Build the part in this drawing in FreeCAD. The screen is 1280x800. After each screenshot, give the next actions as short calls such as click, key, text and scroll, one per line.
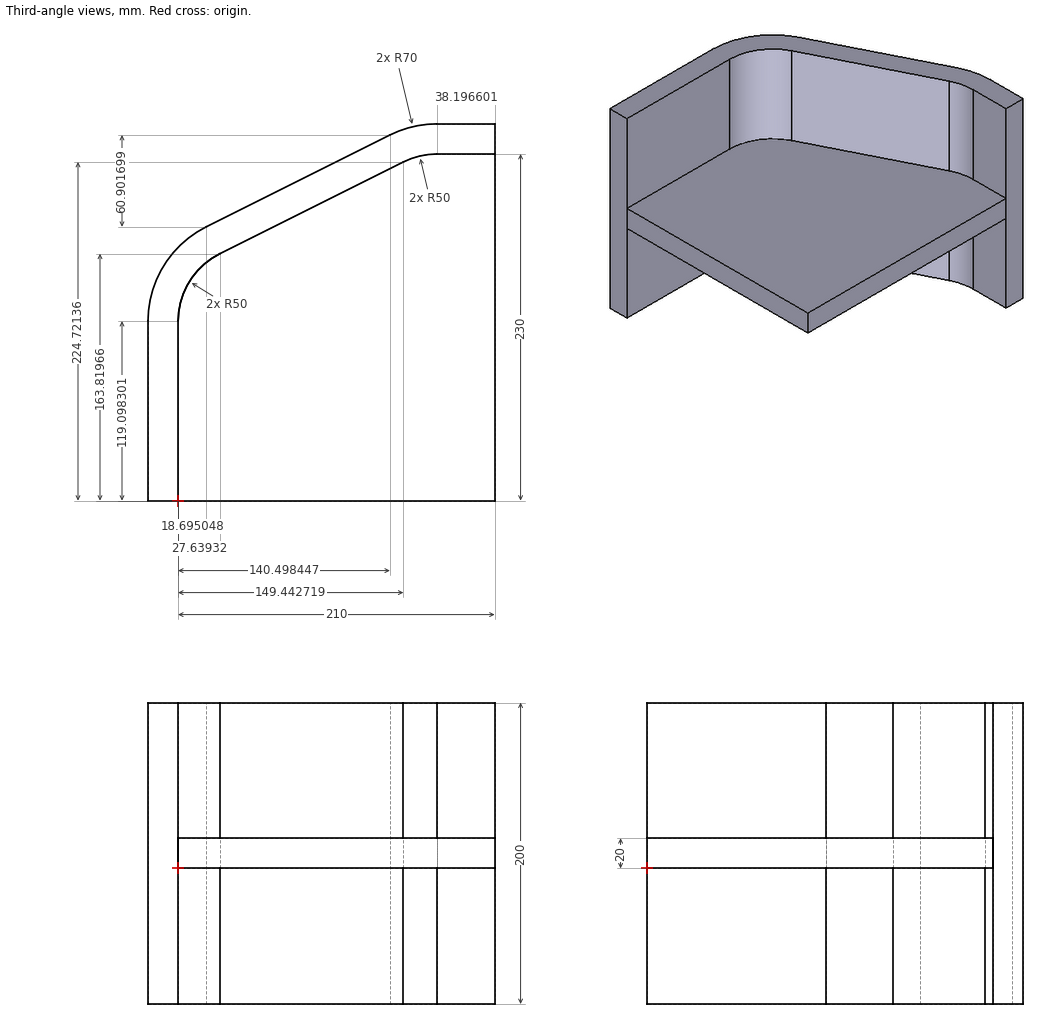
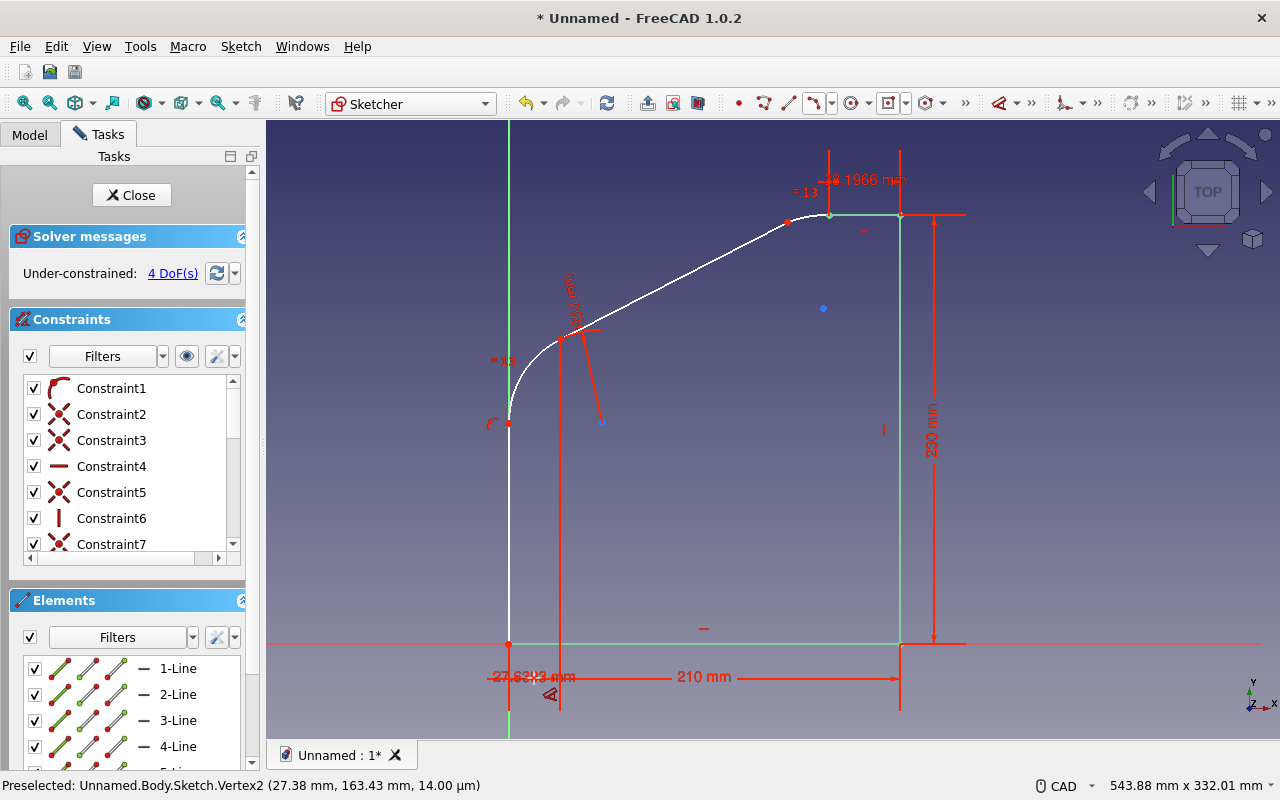
click(509, 490)
click(475, 534)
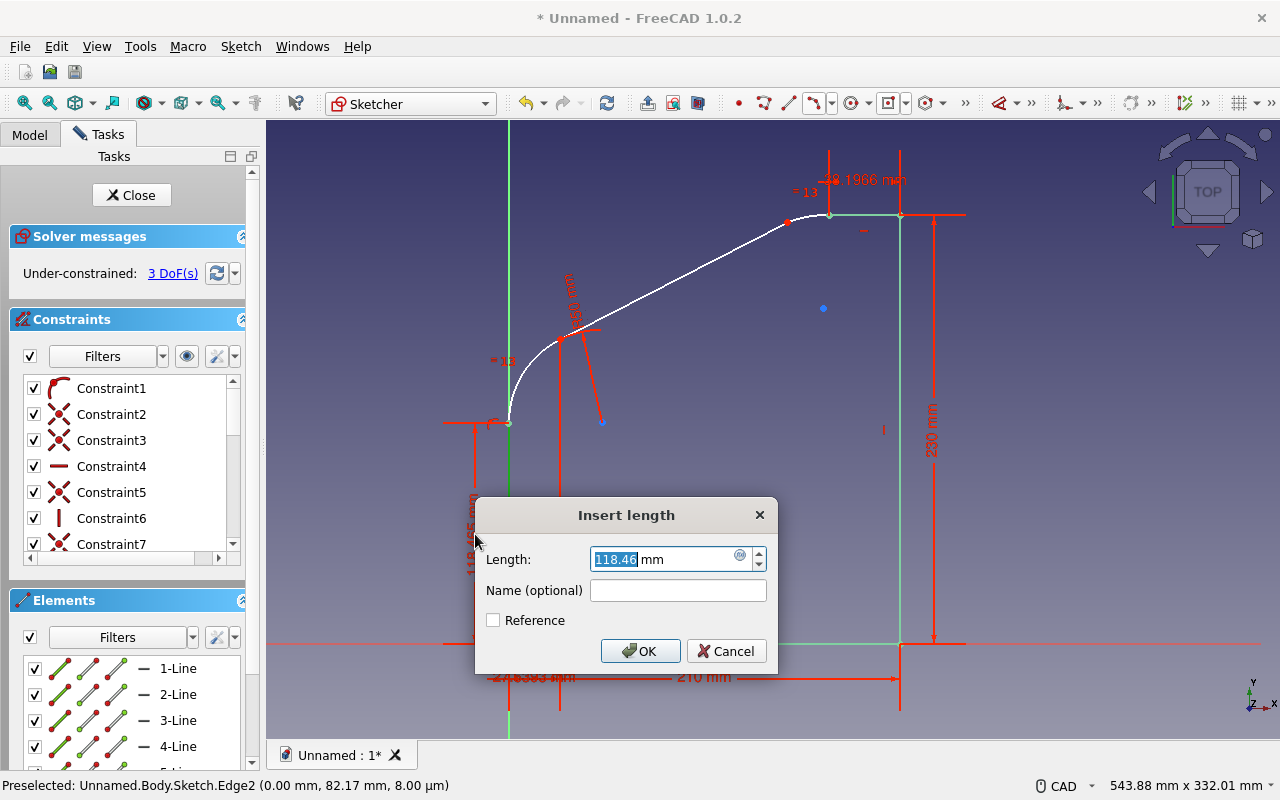
text(119.098301)
key(Return)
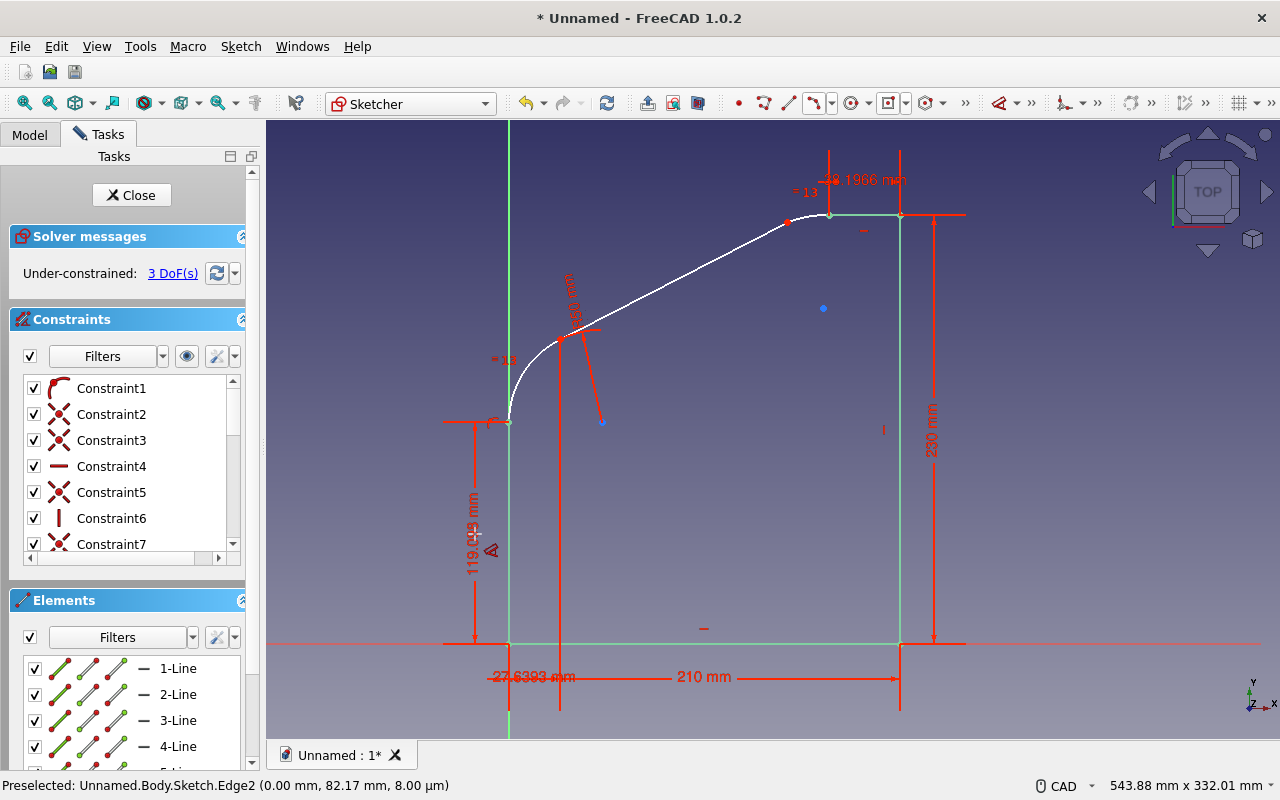
click(788, 223)
click(475, 433)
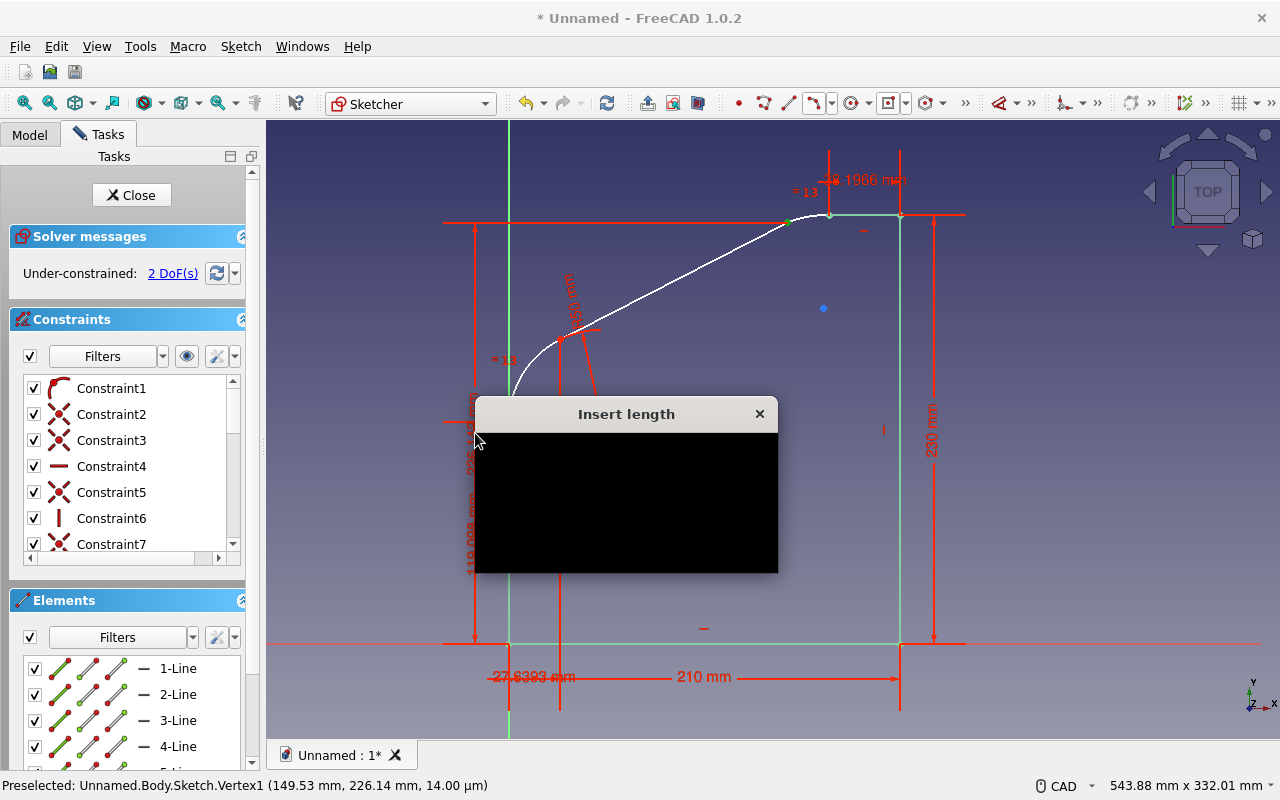
text(224.72136)
key(Return)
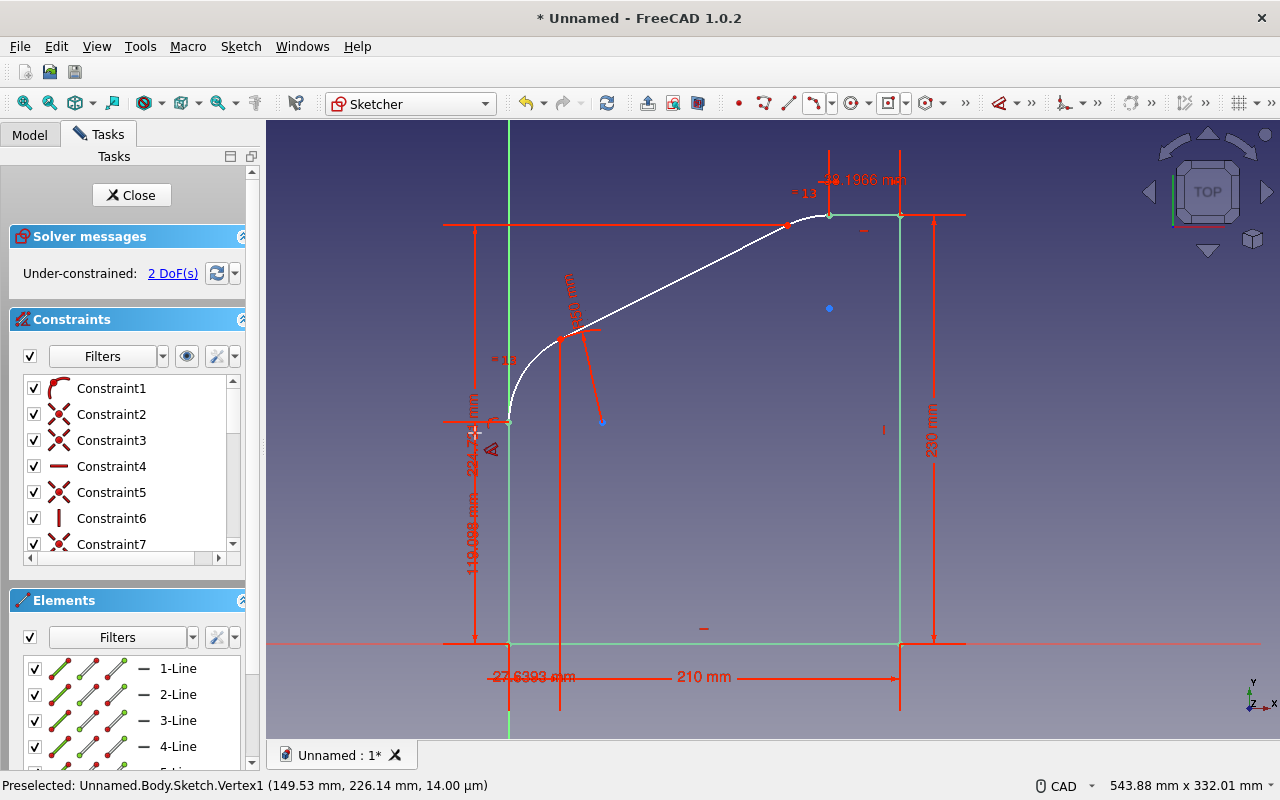
click(560, 340)
click(475, 492)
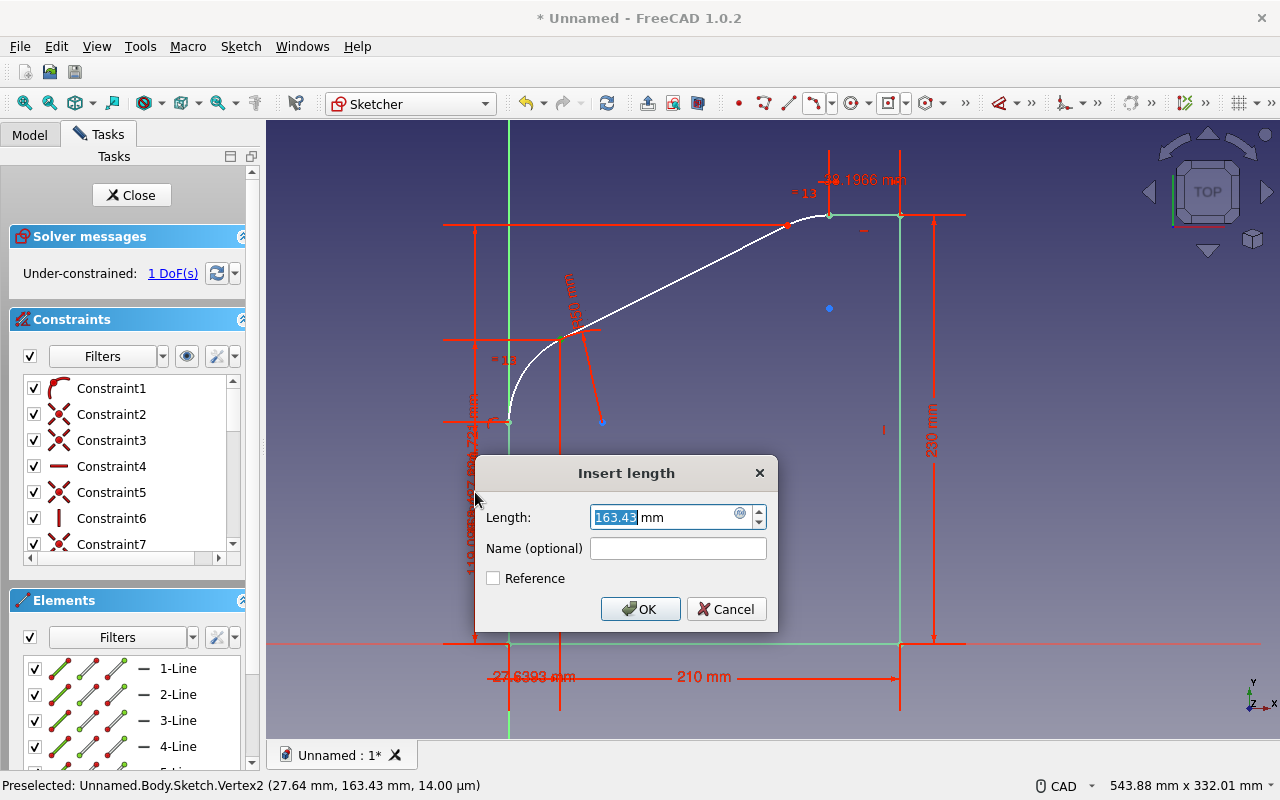
text(163.81966)
key(Return)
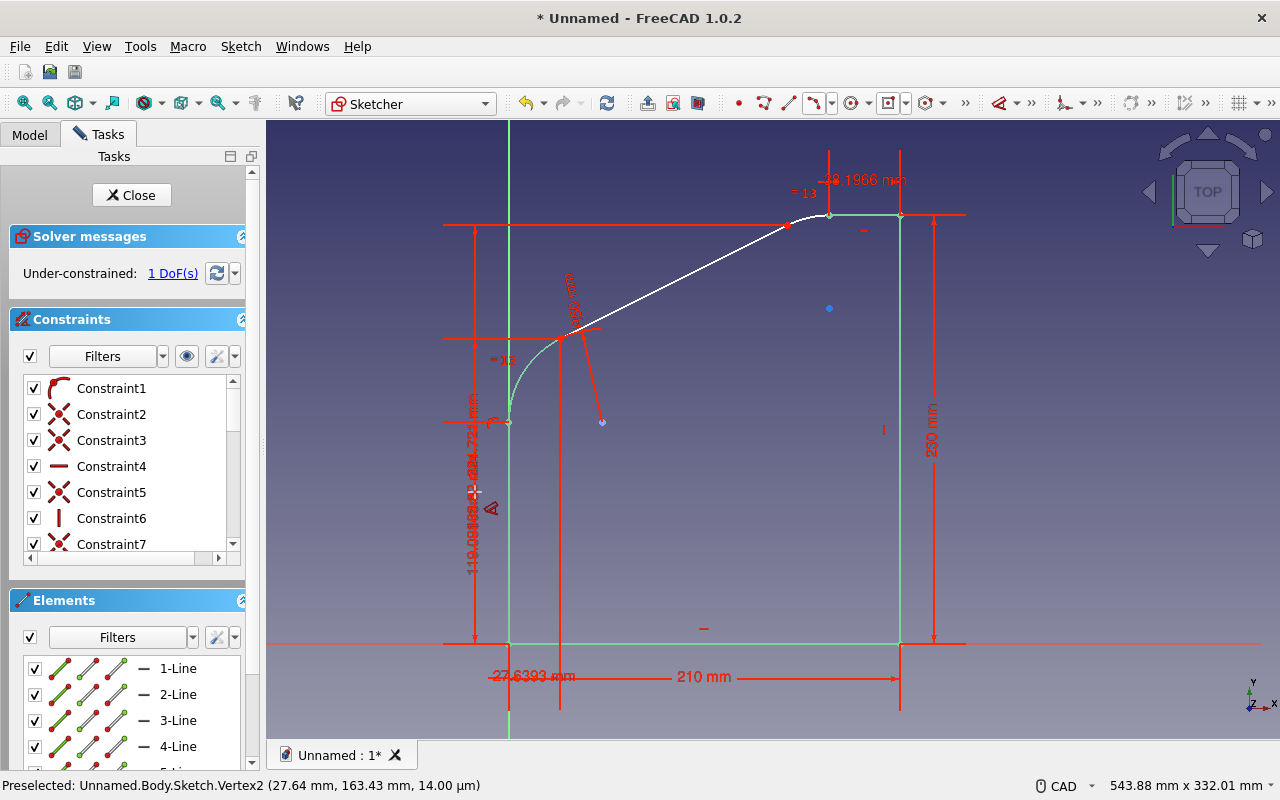
click(788, 225)
click(648, 191)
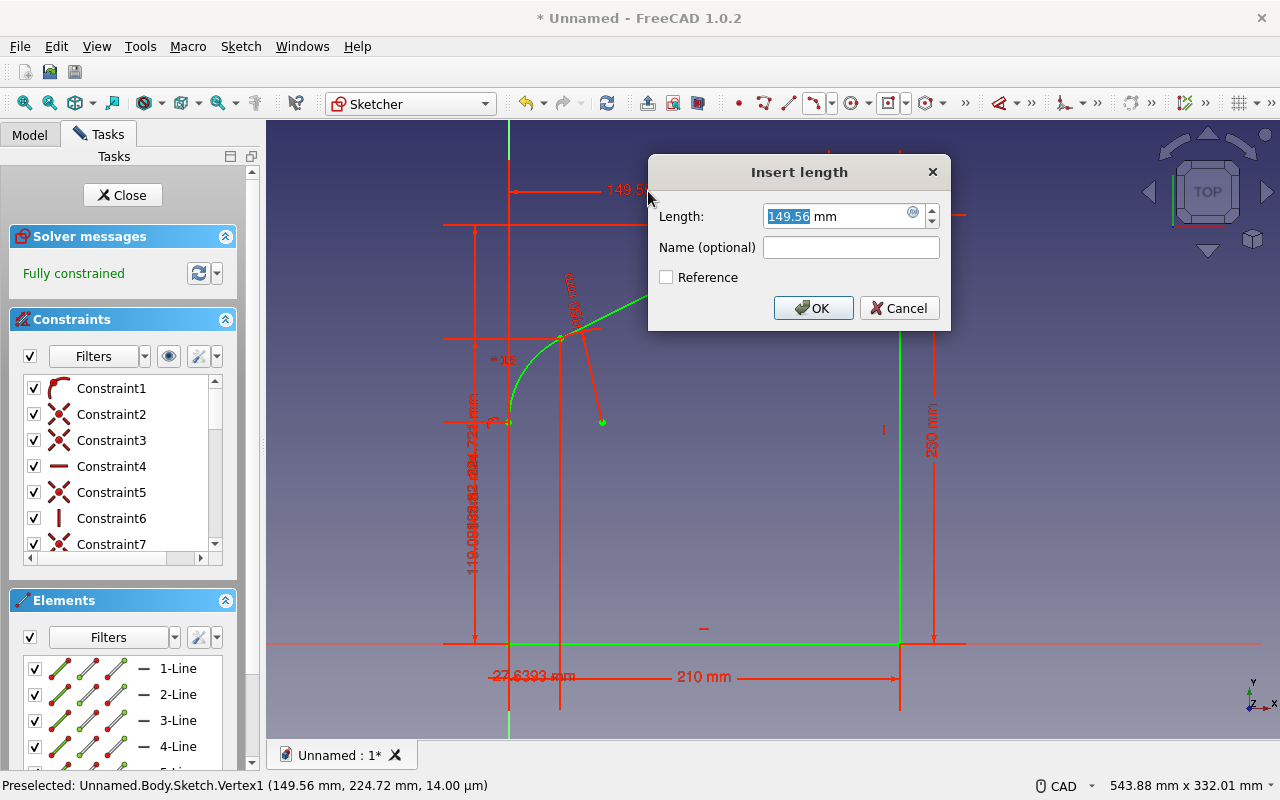
text(149.442719)
key(Return)
key(Escape)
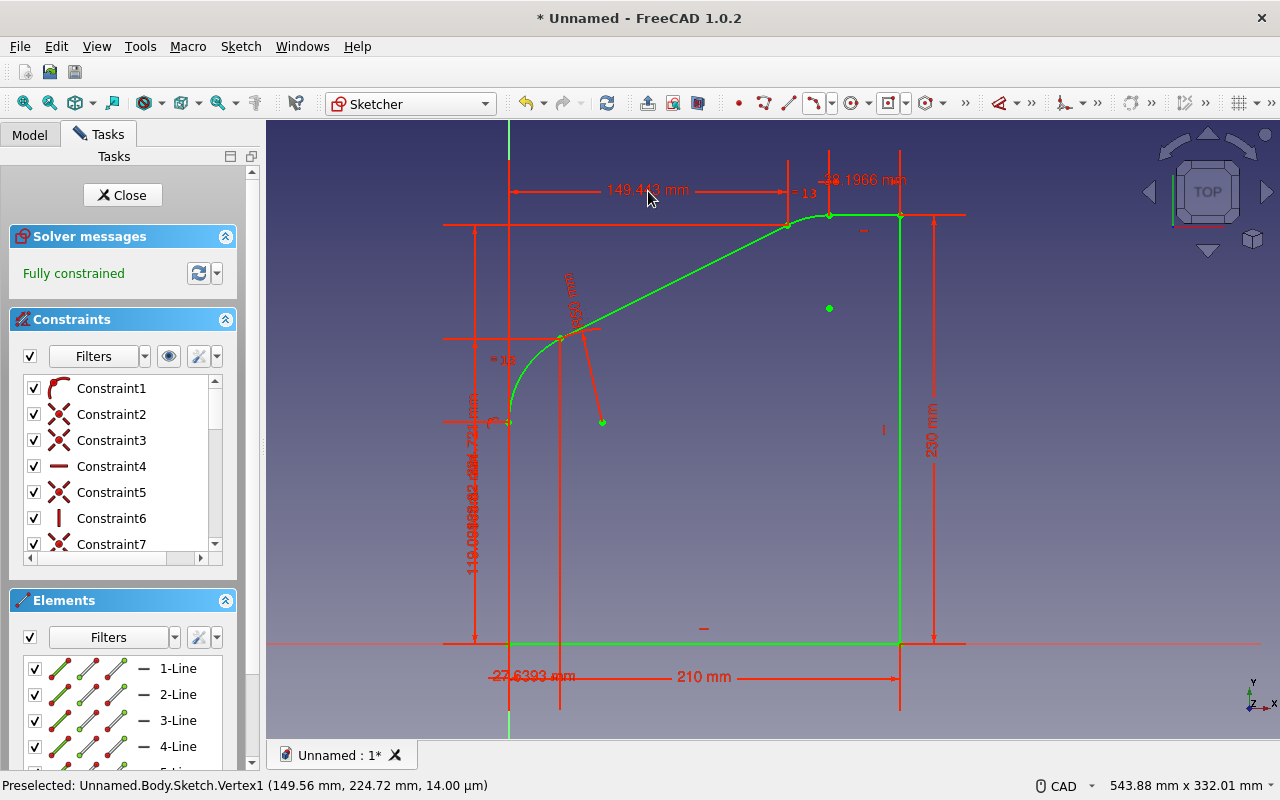
click(123, 195)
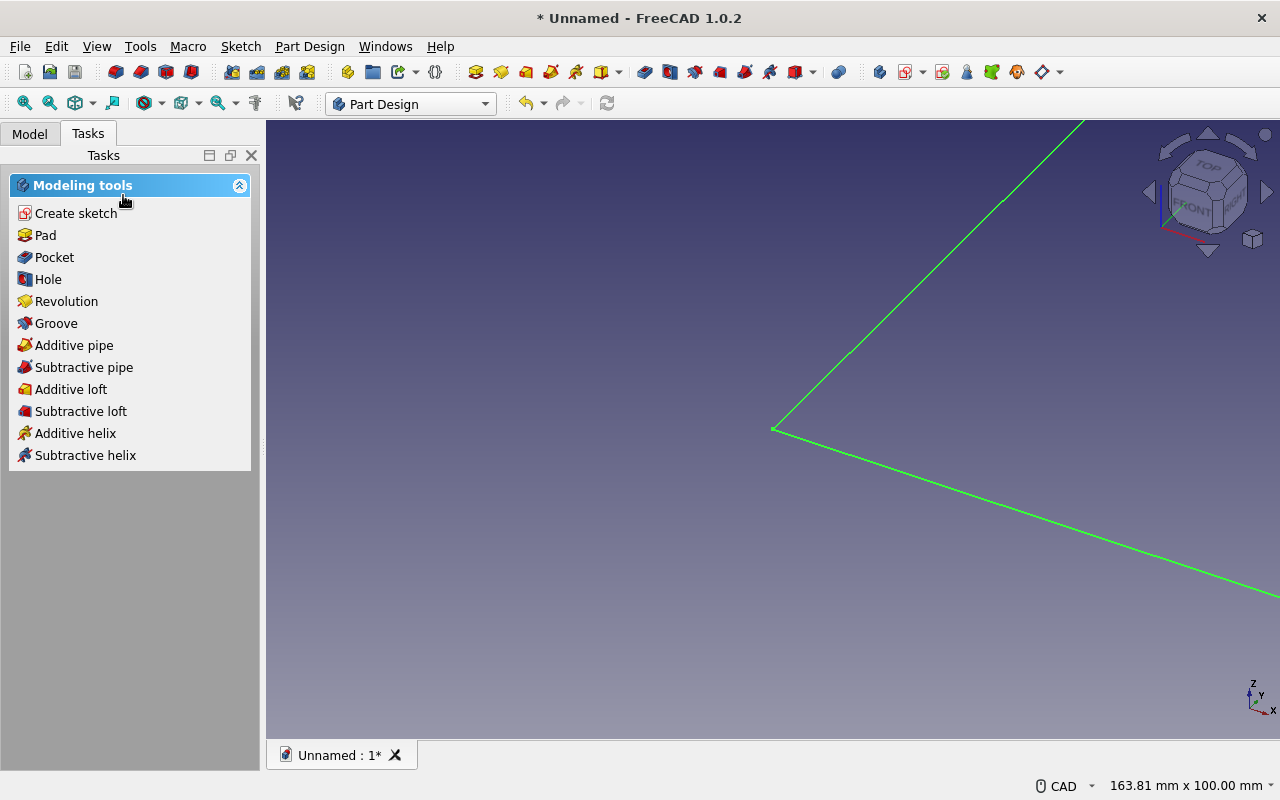
click(476, 72)